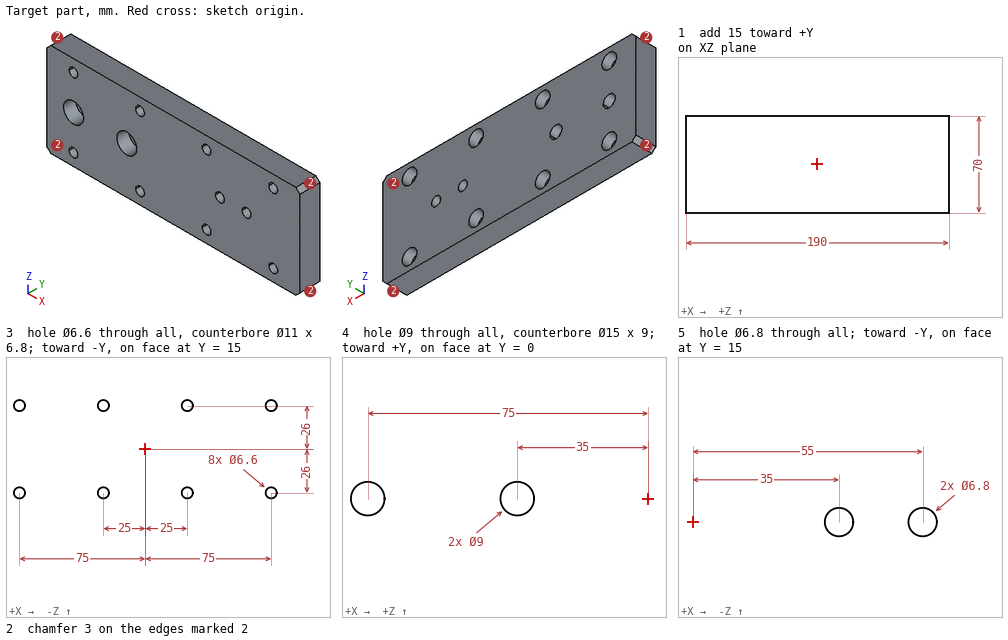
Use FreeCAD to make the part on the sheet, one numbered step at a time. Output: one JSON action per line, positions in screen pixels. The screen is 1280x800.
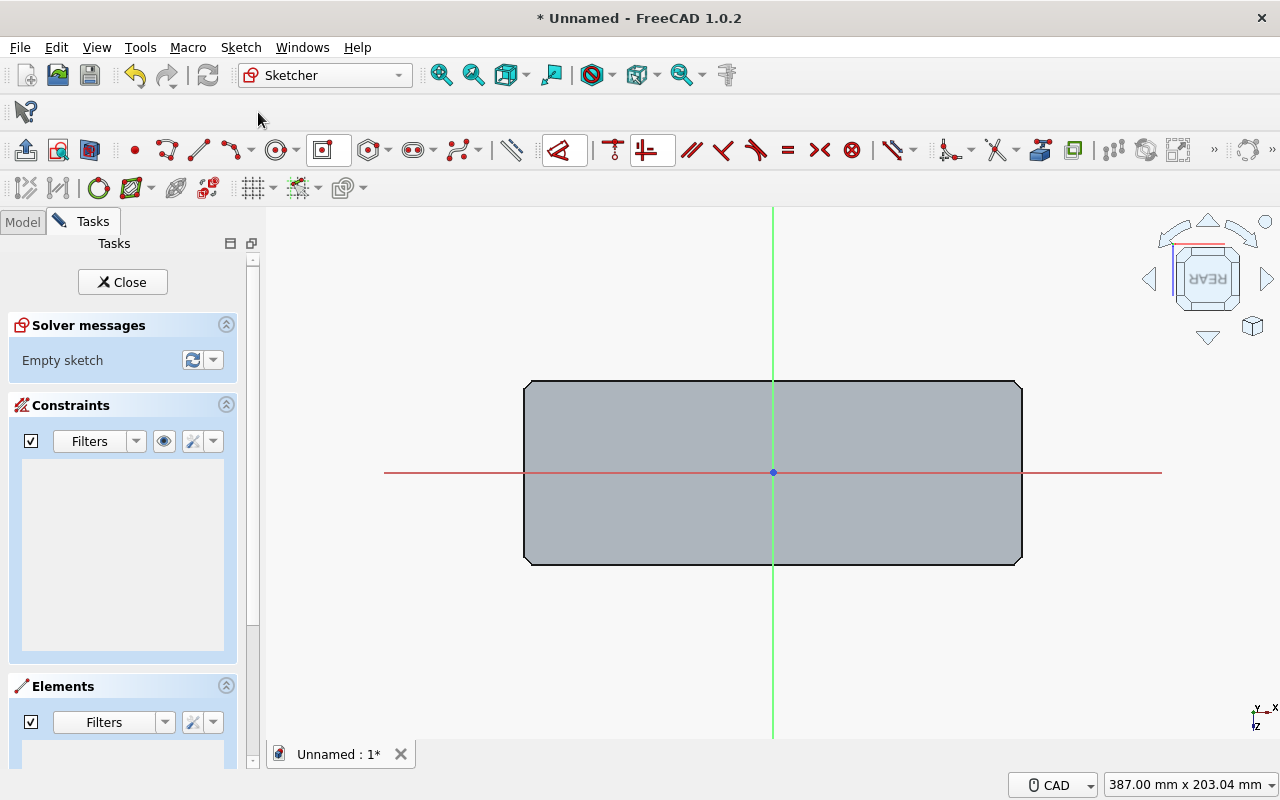
{"action": "scroll", "coordinate": [912, 473], "scroll_direction": "up", "scroll_amount": 2}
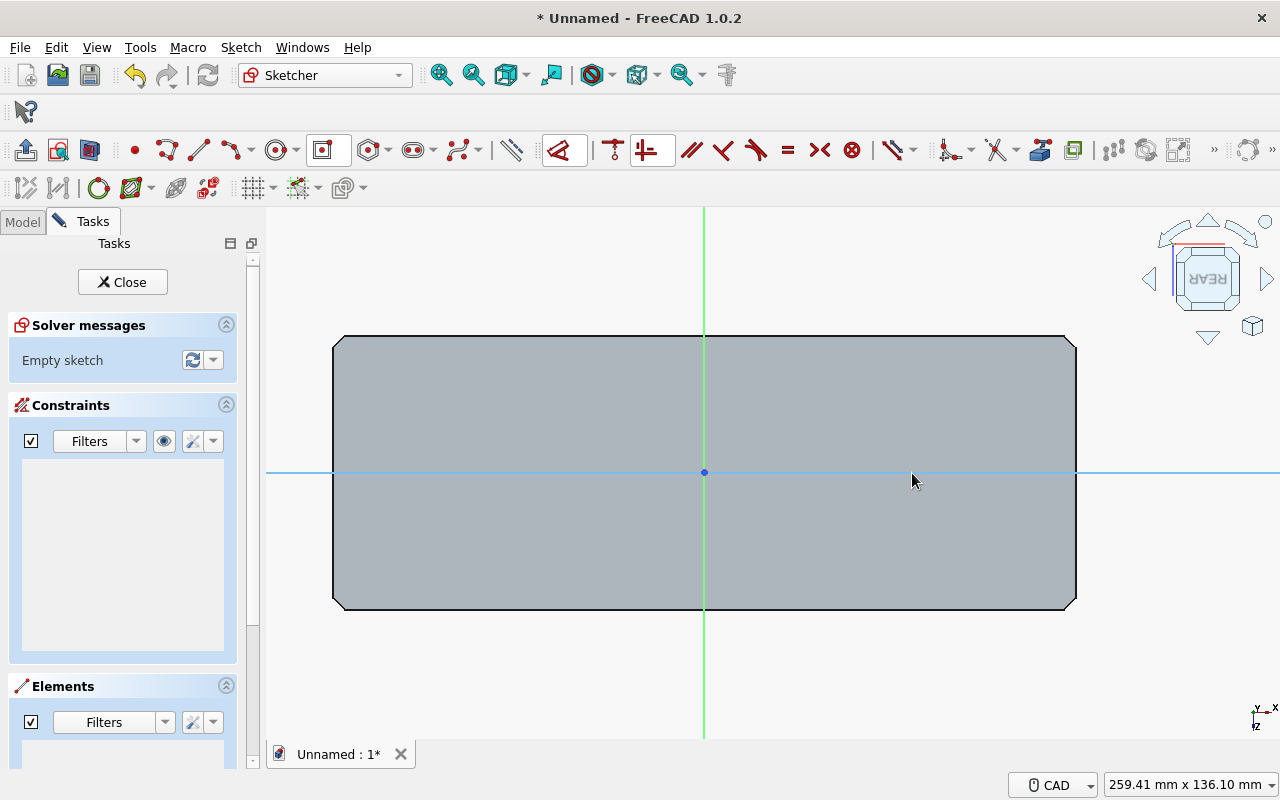
{"action": "left_click", "coordinate": [276, 150]}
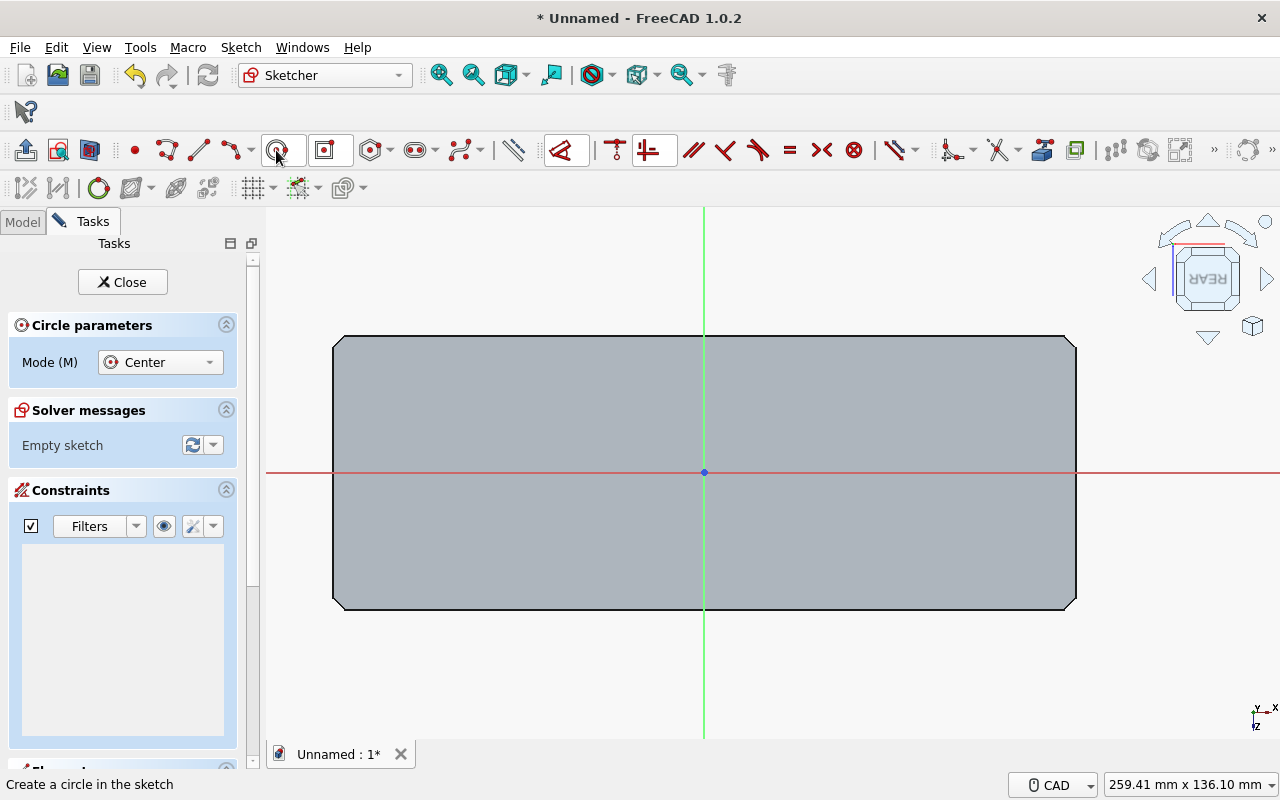
{"action": "scroll", "coordinate": [997, 574], "scroll_direction": "up", "scroll_amount": 3}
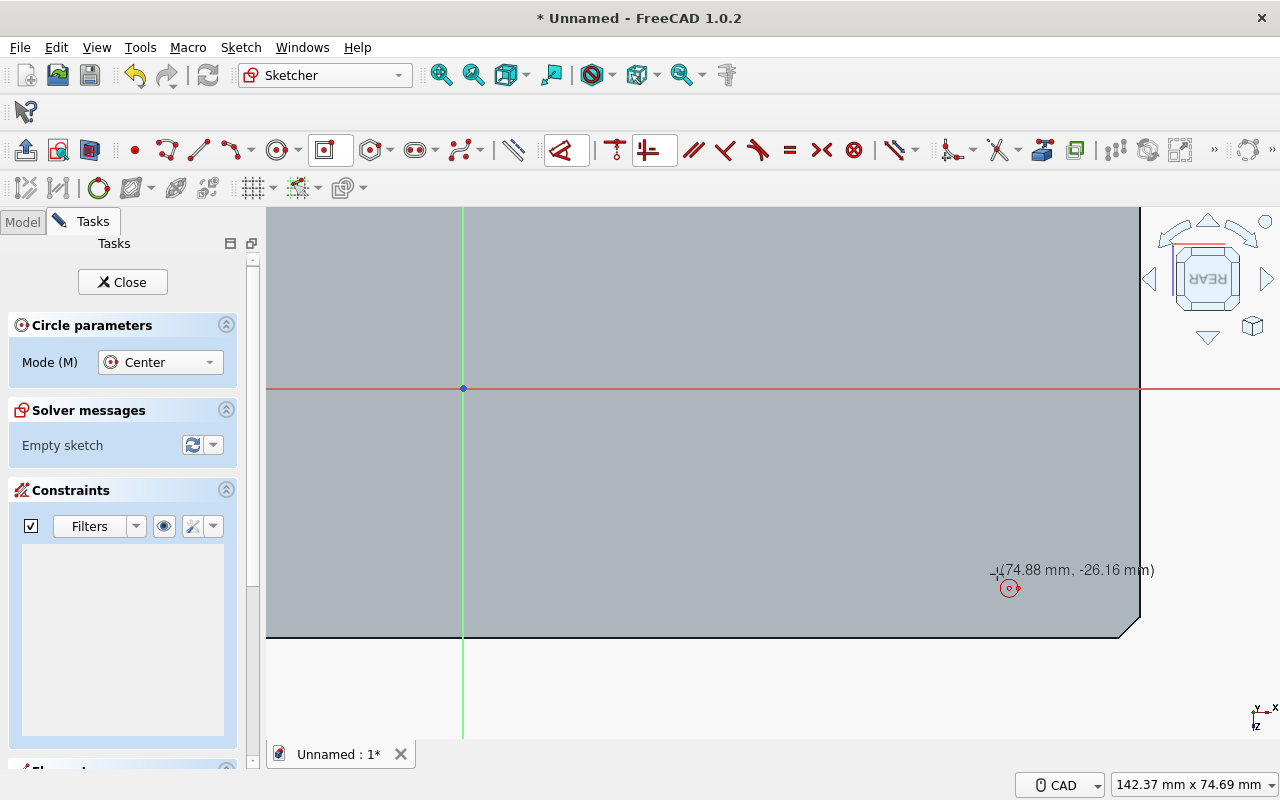
{"action": "left_click", "coordinate": [997, 574]}
{"action": "mouse_move", "coordinate": [1014, 558]}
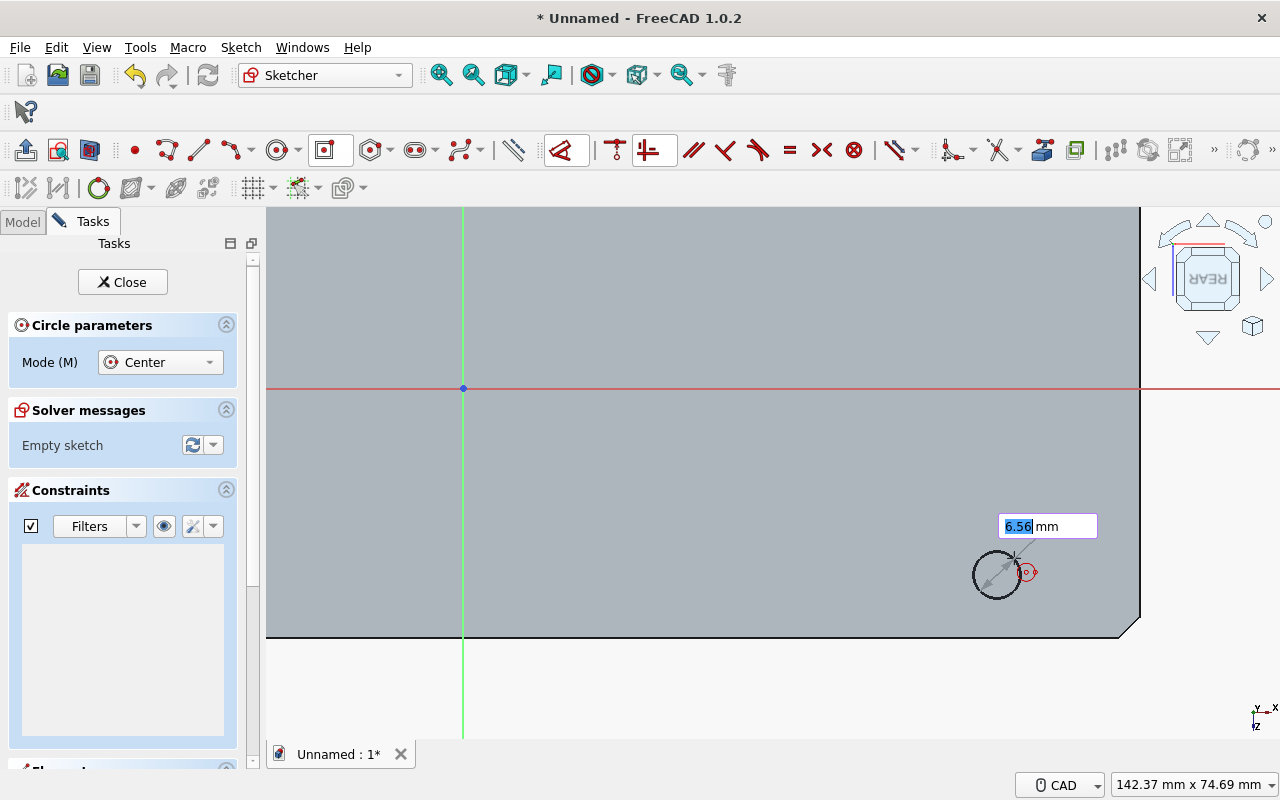
{"action": "type", "text": "6.6"}
{"action": "key", "text": "Return"}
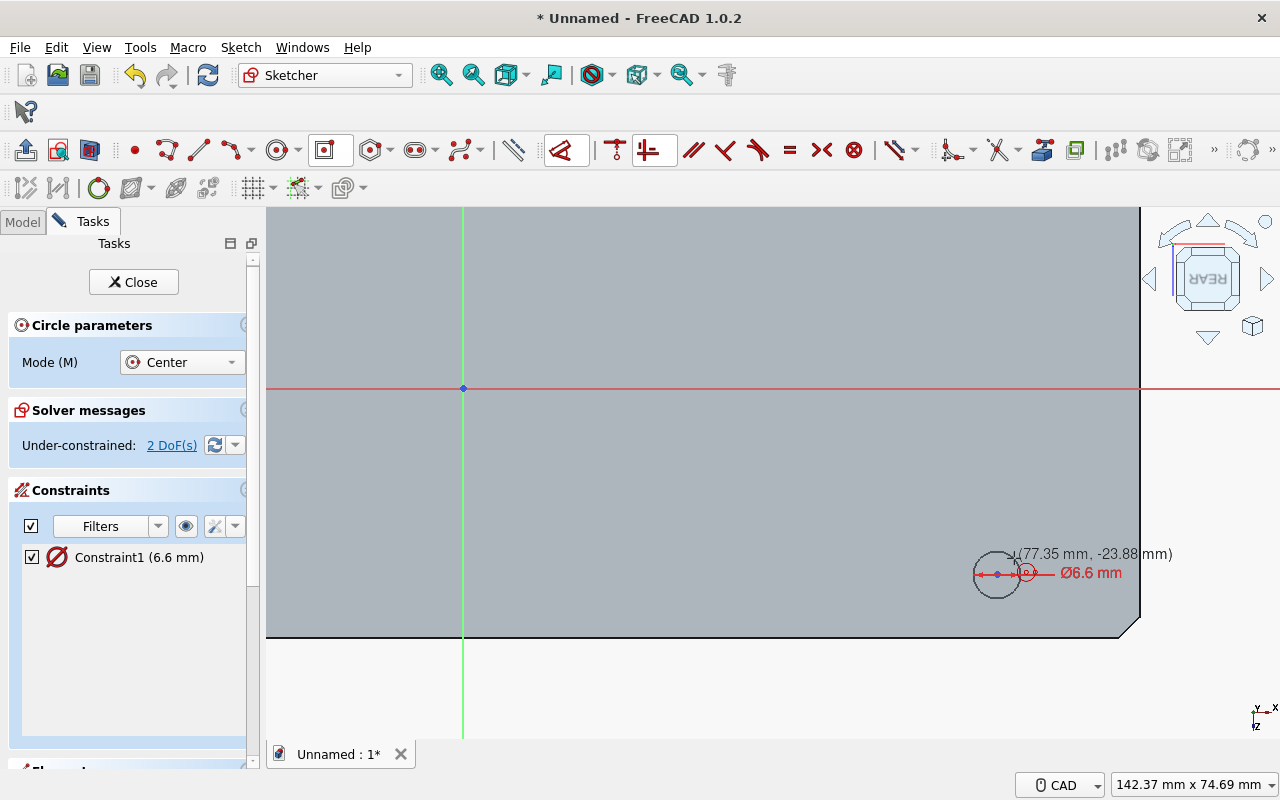
{"action": "left_click", "coordinate": [641, 574]}
{"action": "mouse_move", "coordinate": [658, 558]}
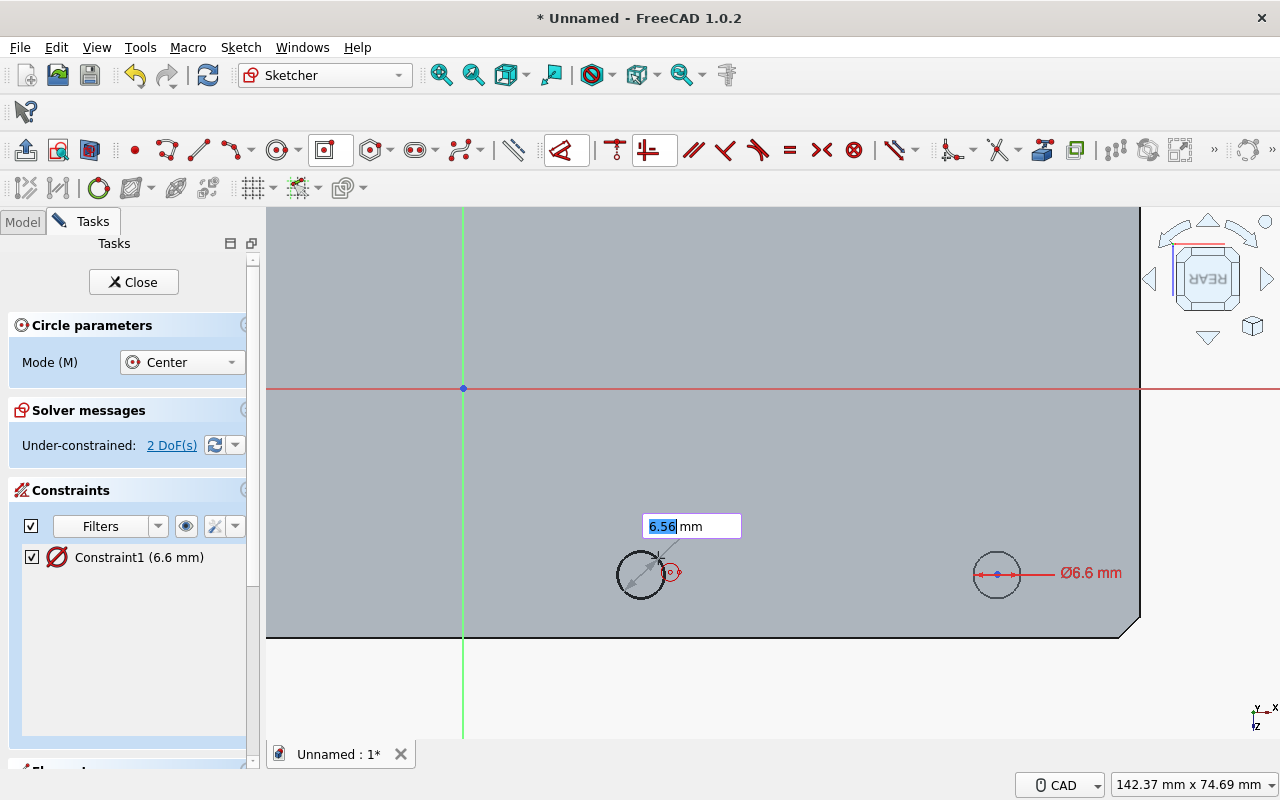
{"action": "type", "text": "6.6"}
{"action": "key", "text": "Return"}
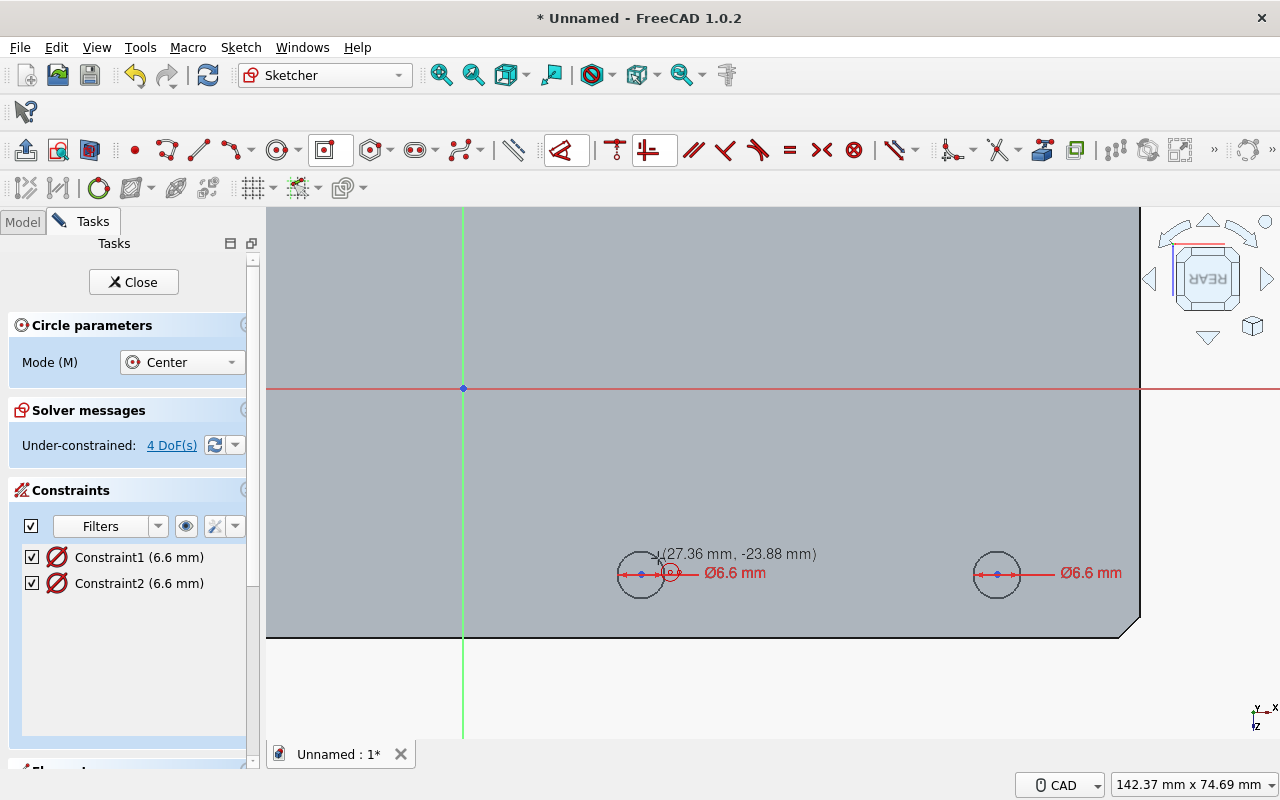
{"action": "scroll", "coordinate": [998, 575], "scroll_direction": "down", "scroll_amount": 3}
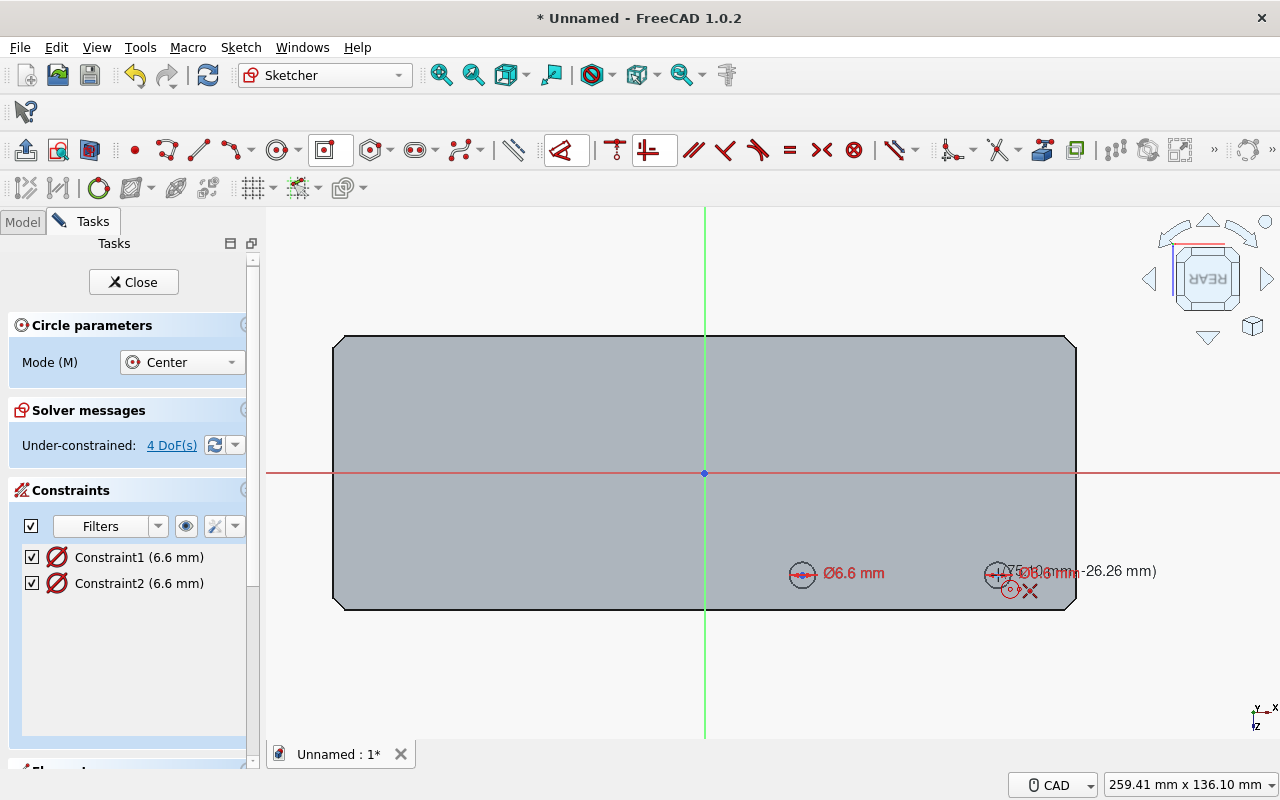
{"action": "scroll", "coordinate": [607, 575], "scroll_direction": "up", "scroll_amount": 3}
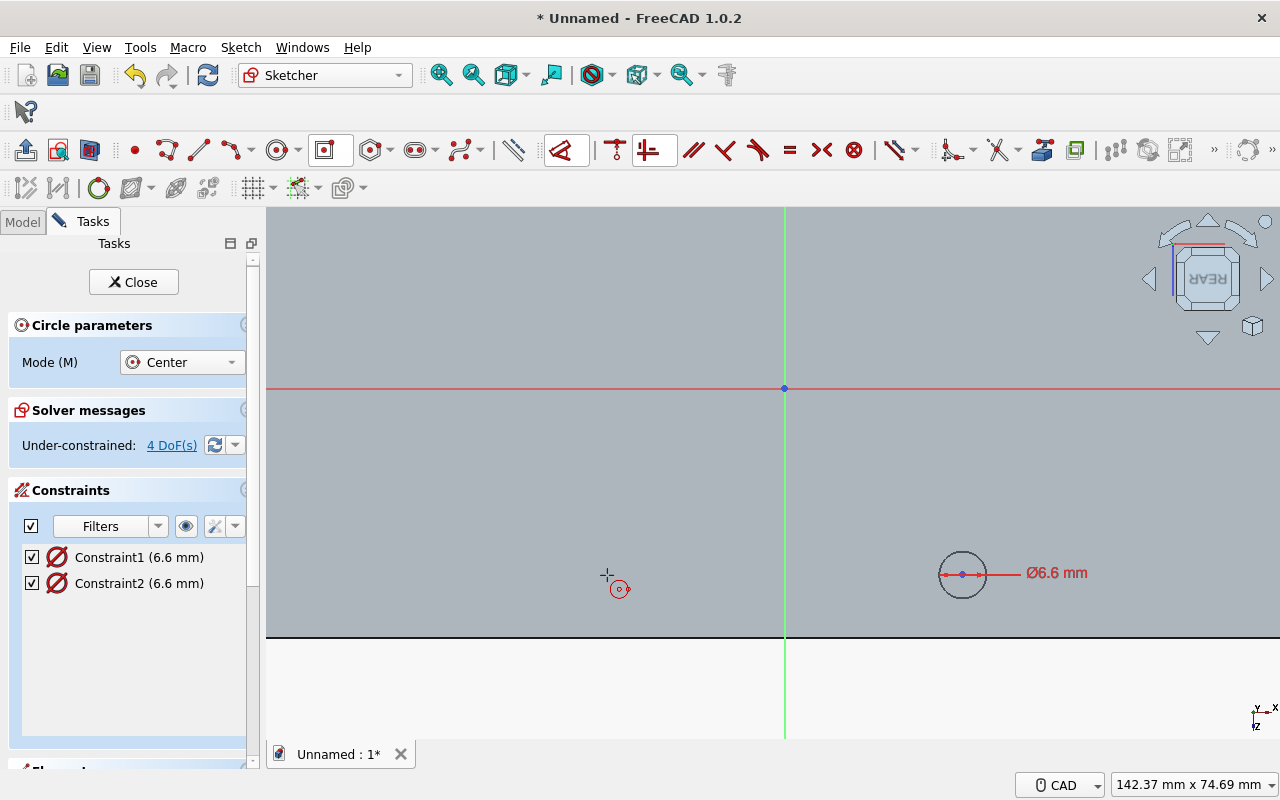
{"action": "left_click", "coordinate": [607, 574]}
{"action": "mouse_move", "coordinate": [623, 558]}